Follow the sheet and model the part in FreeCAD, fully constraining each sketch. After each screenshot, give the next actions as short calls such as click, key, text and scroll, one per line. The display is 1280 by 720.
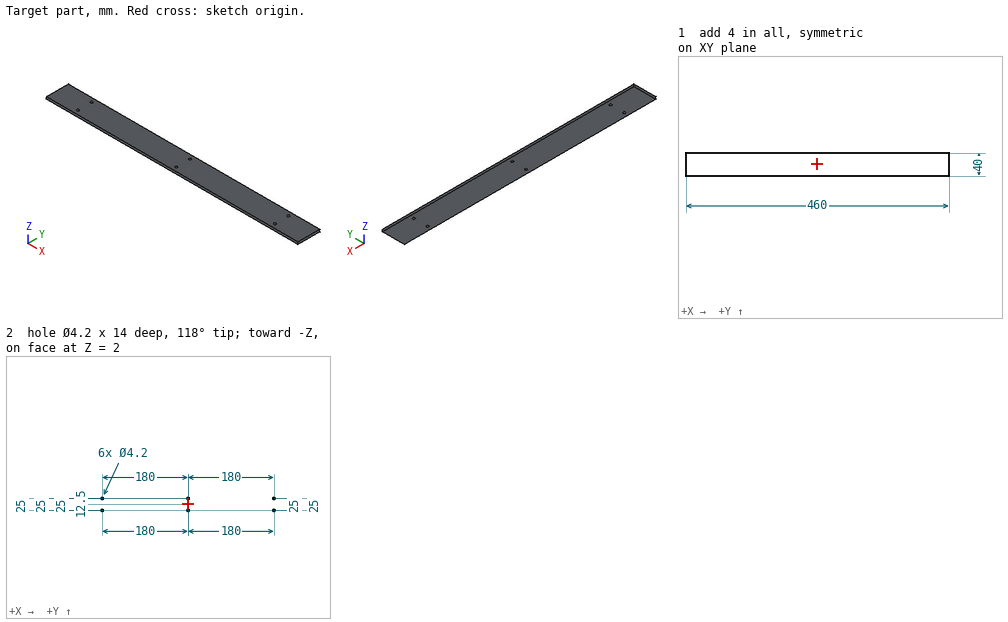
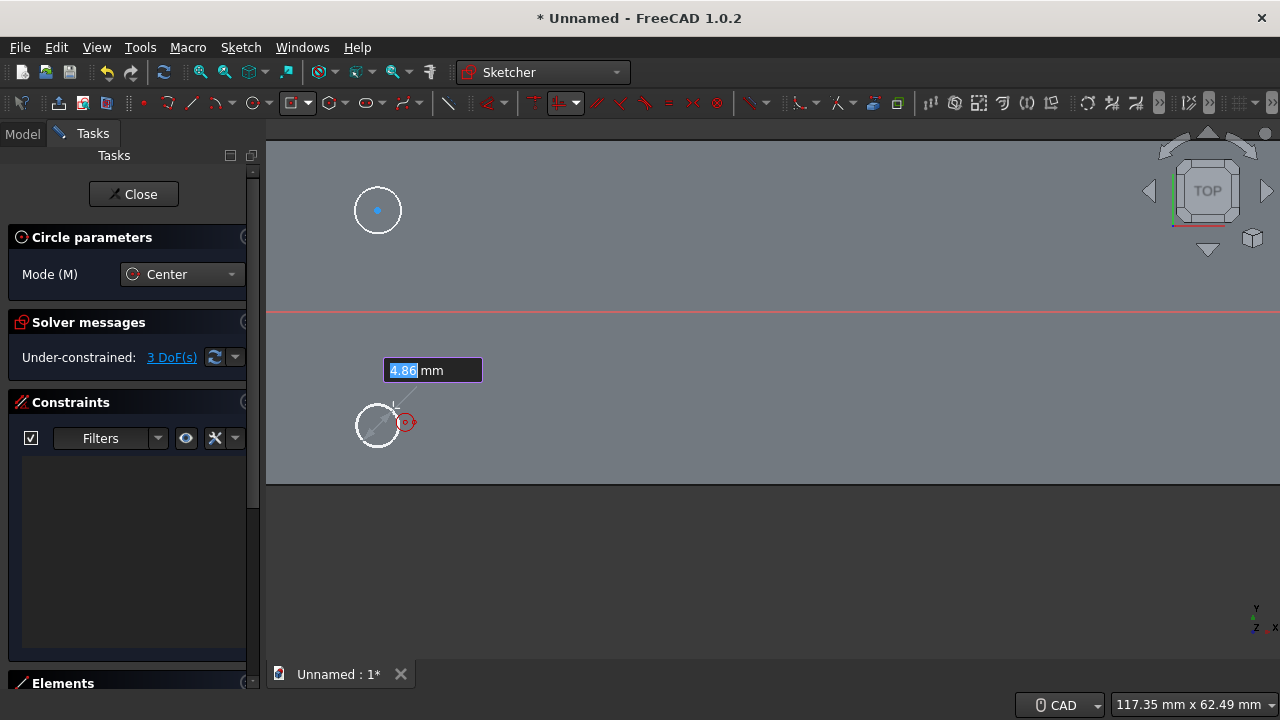
click(392, 408)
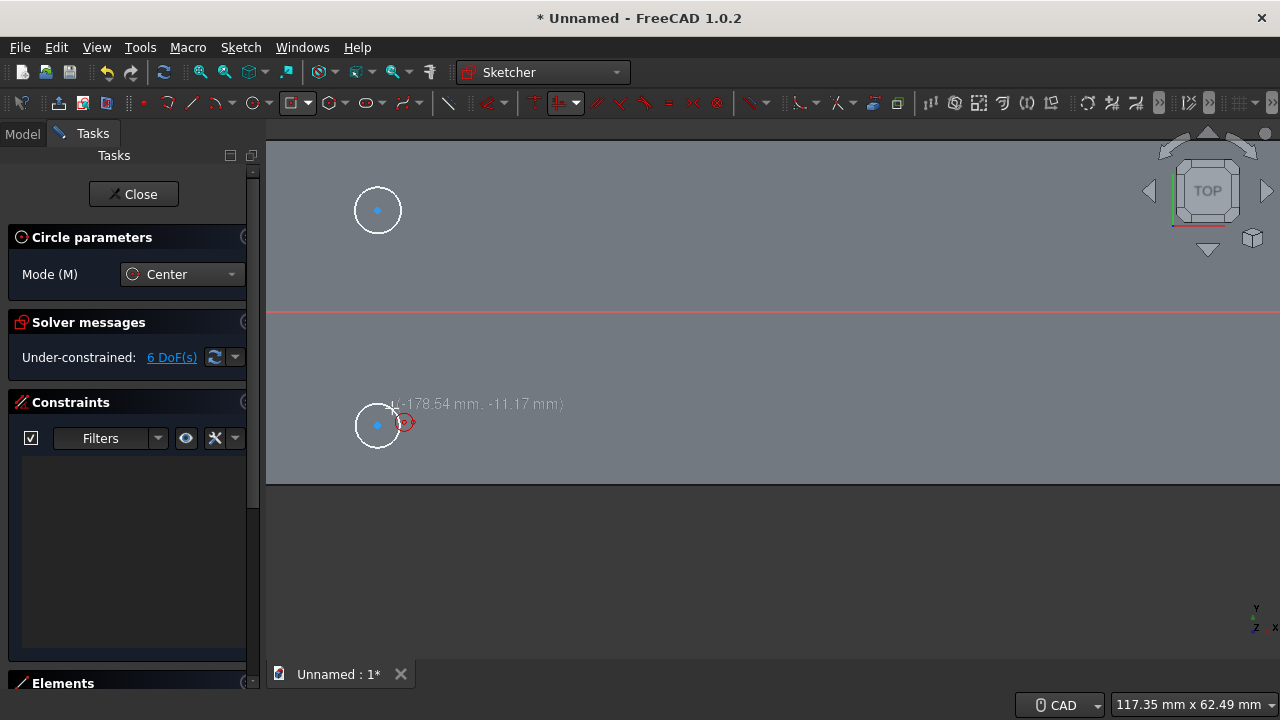
scroll(393, 408, down, 8)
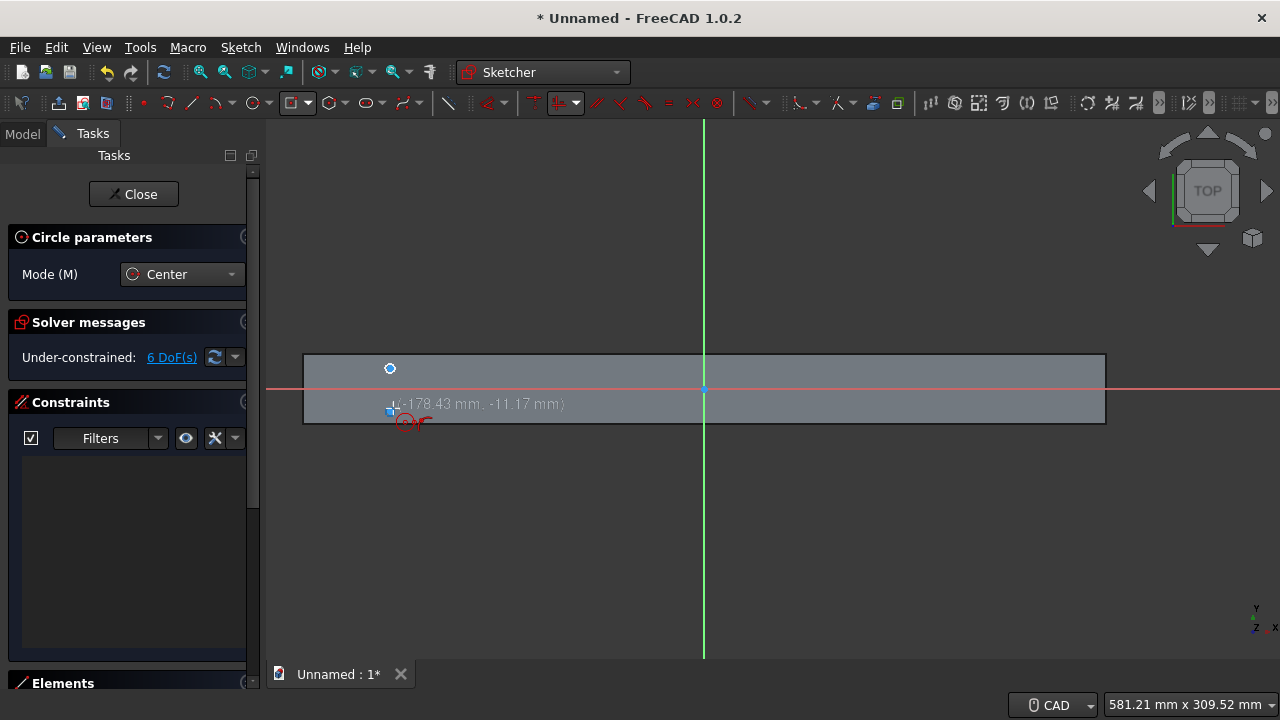
scroll(704, 367, up, 10)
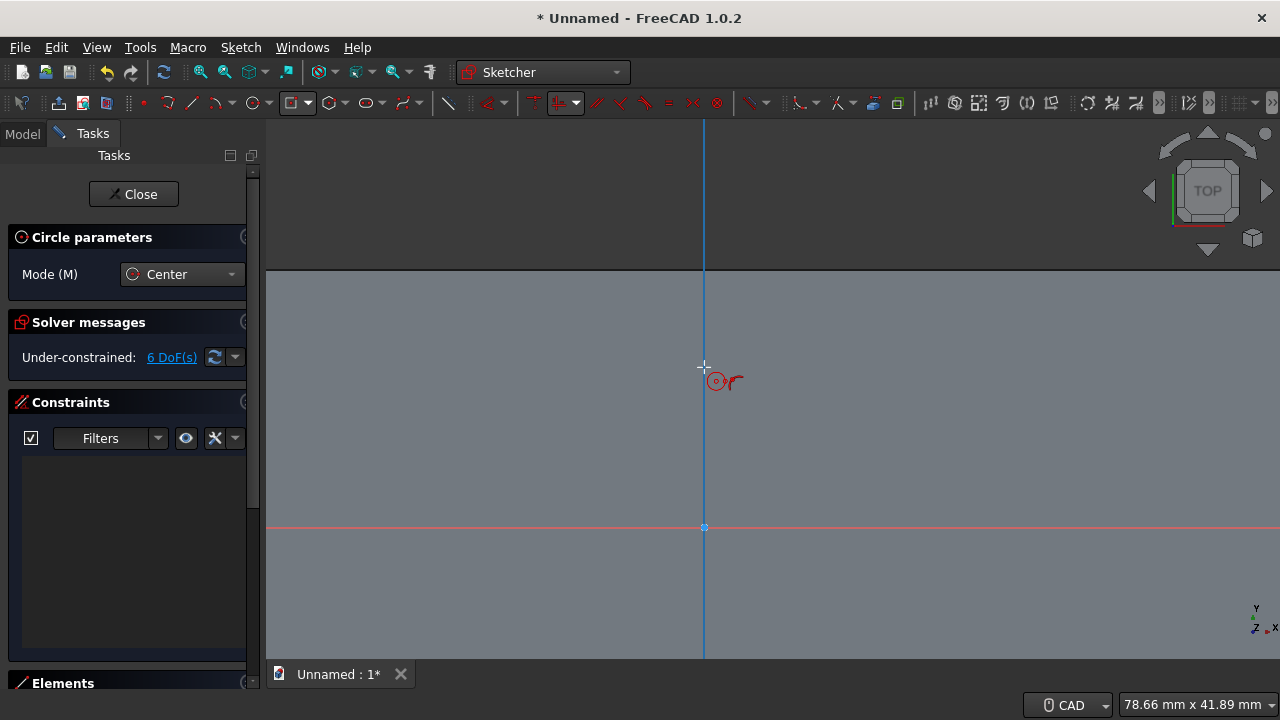
scroll(705, 367, down, 10)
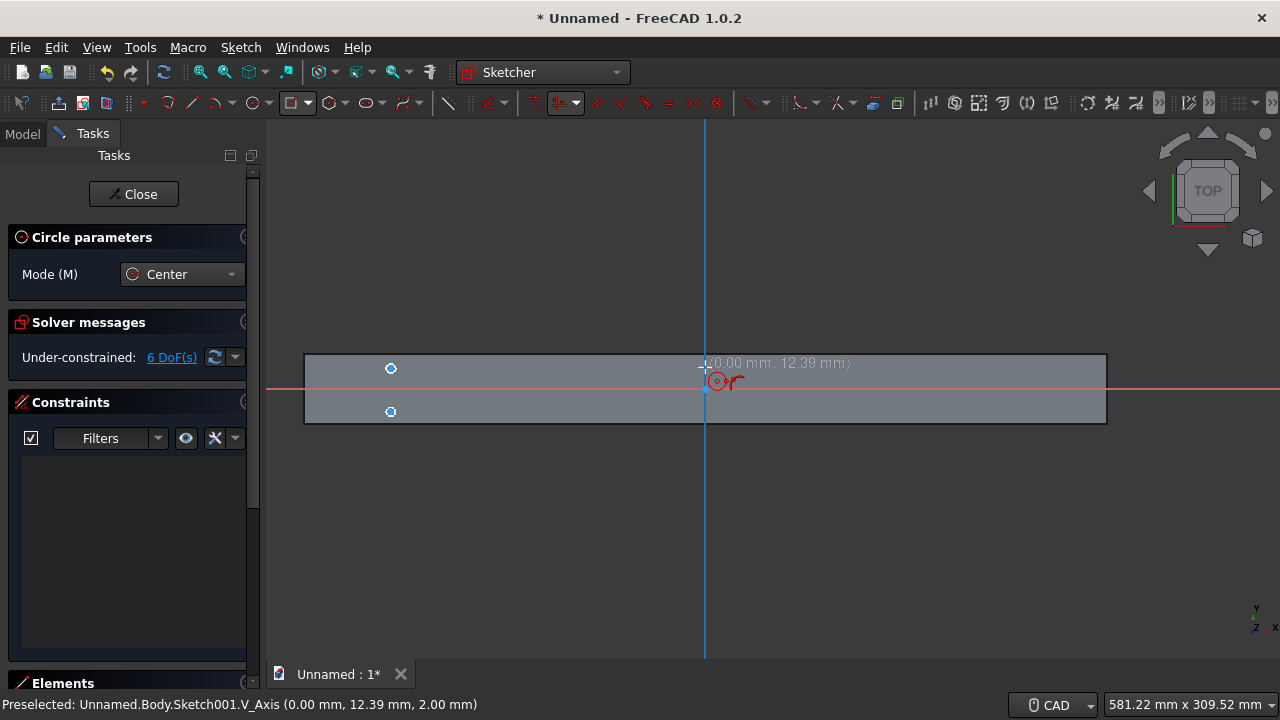
click(705, 367)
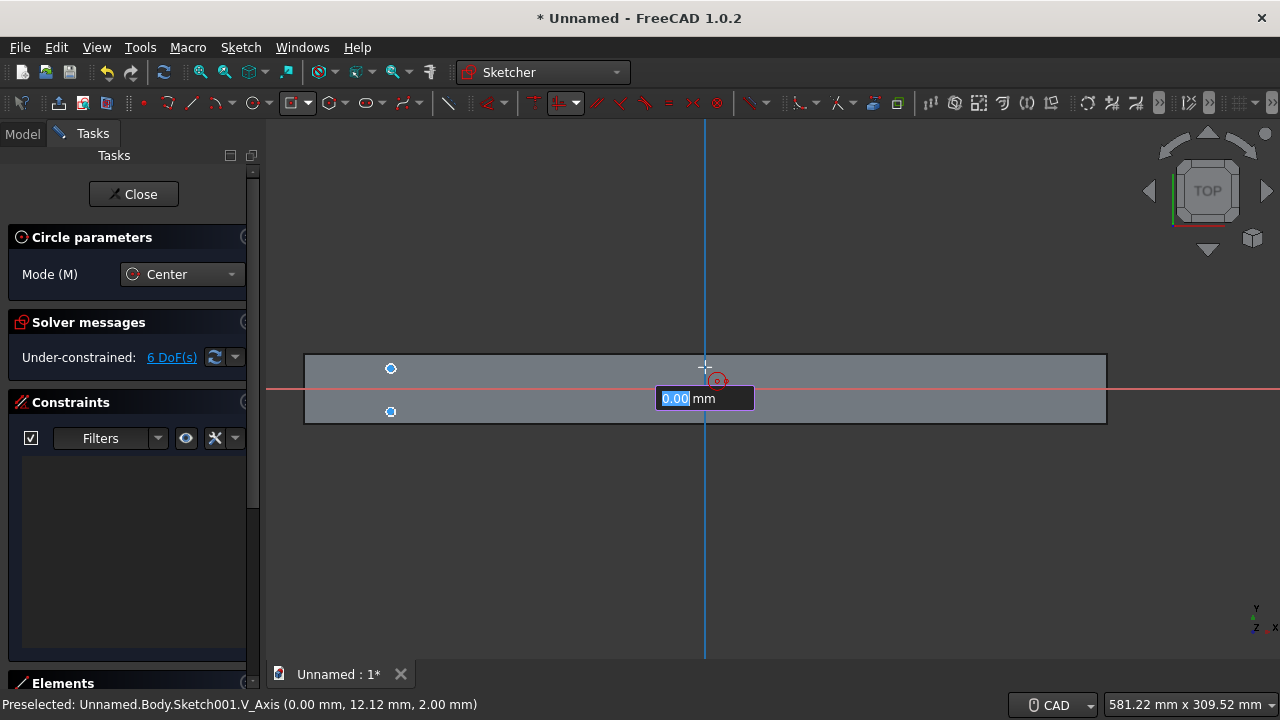
scroll(709, 366, up, 8)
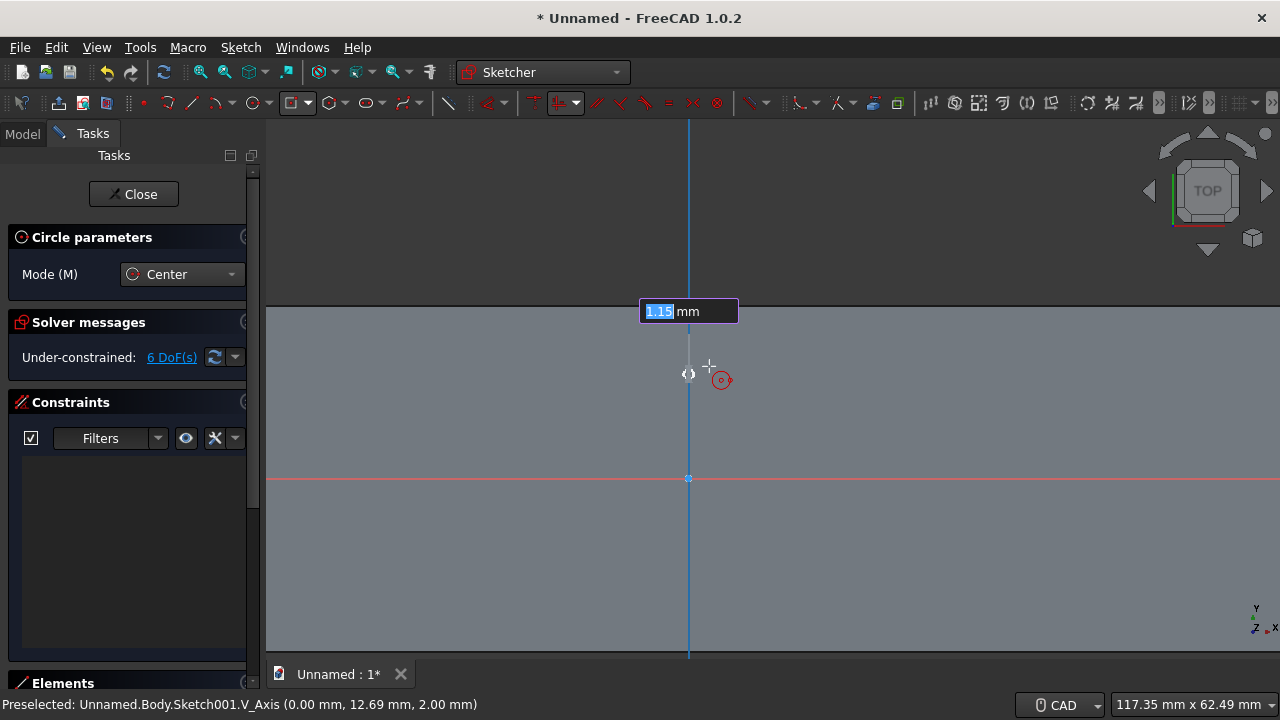
click(706, 365)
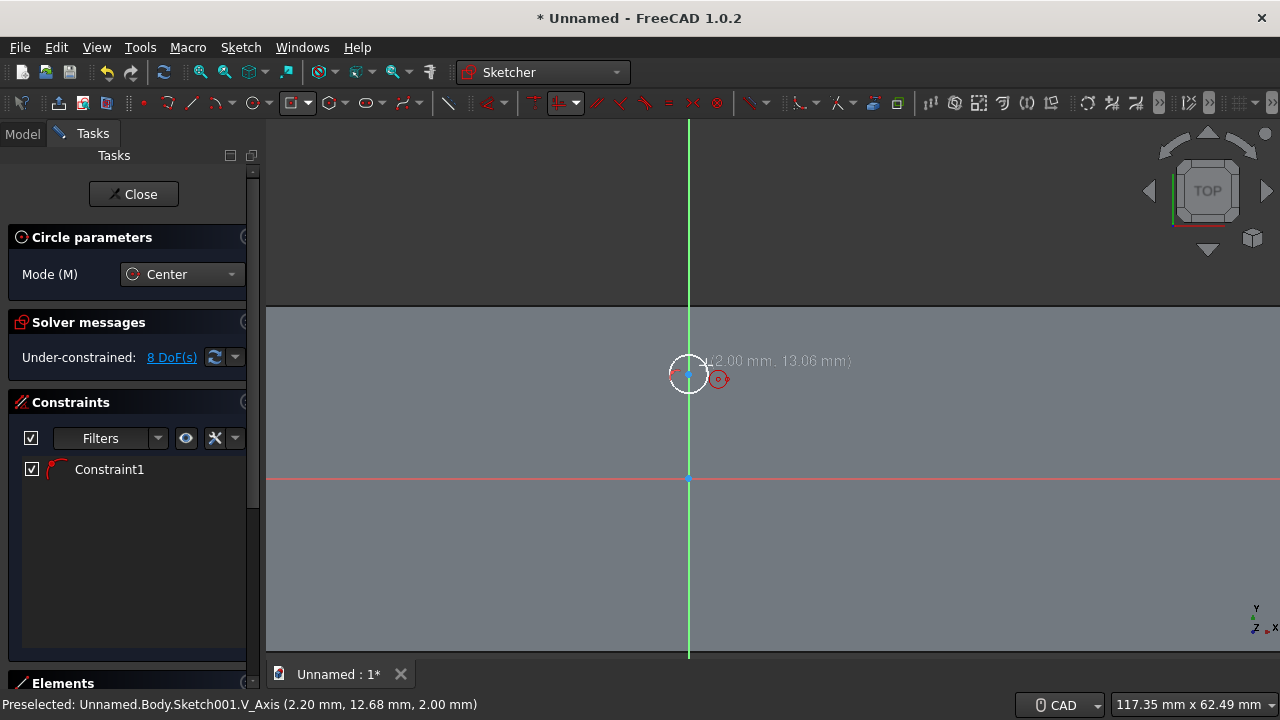
scroll(689, 587, up, 2)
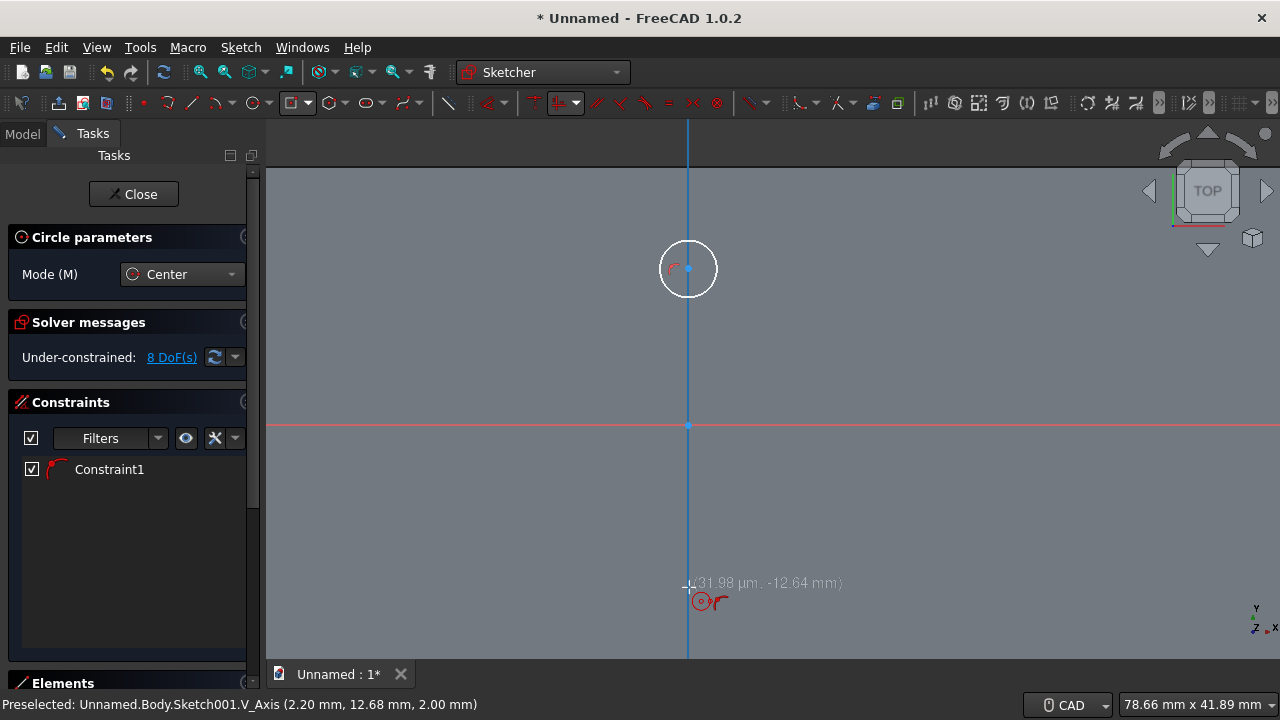
scroll(707, 383, down, 10)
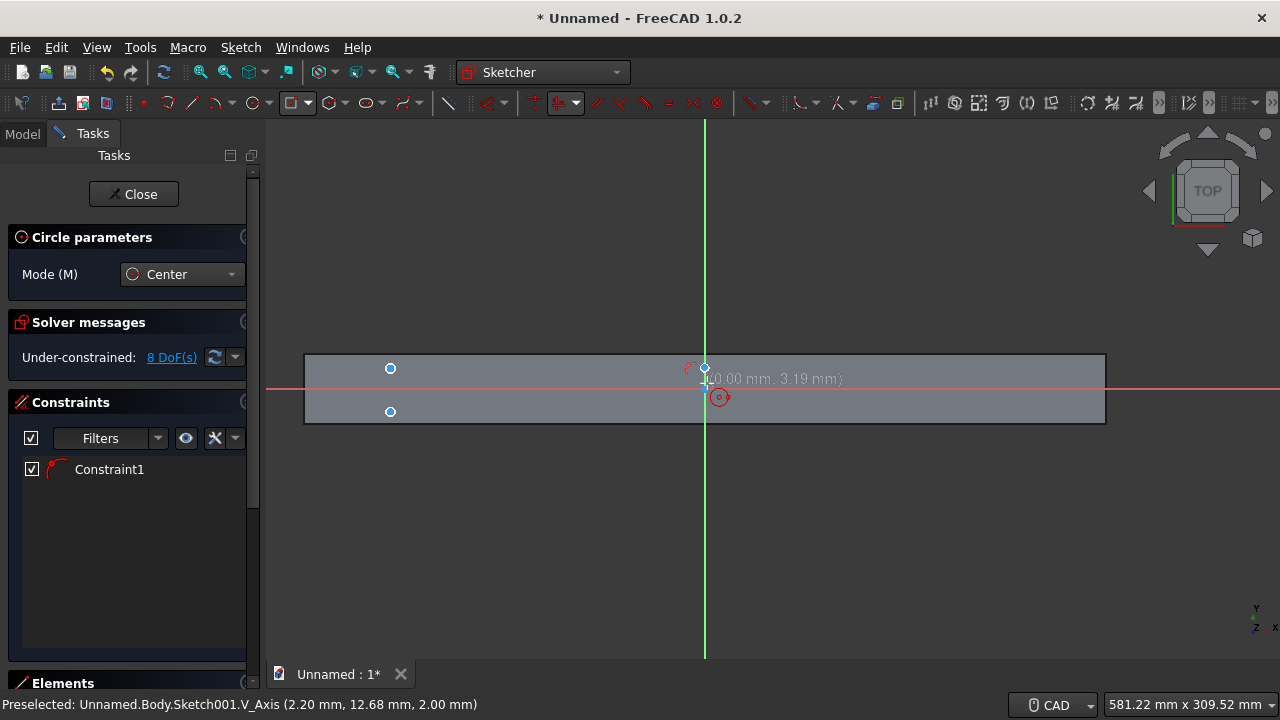
click(705, 411)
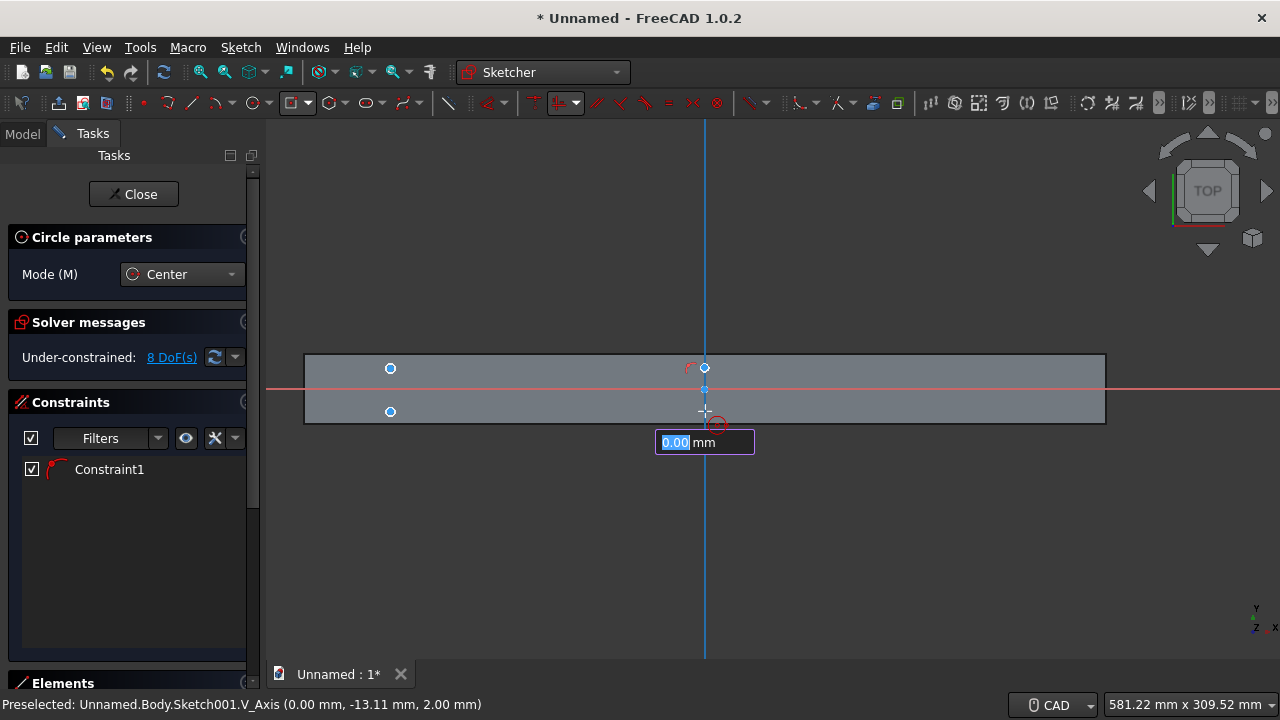
scroll(708, 410, up, 8)